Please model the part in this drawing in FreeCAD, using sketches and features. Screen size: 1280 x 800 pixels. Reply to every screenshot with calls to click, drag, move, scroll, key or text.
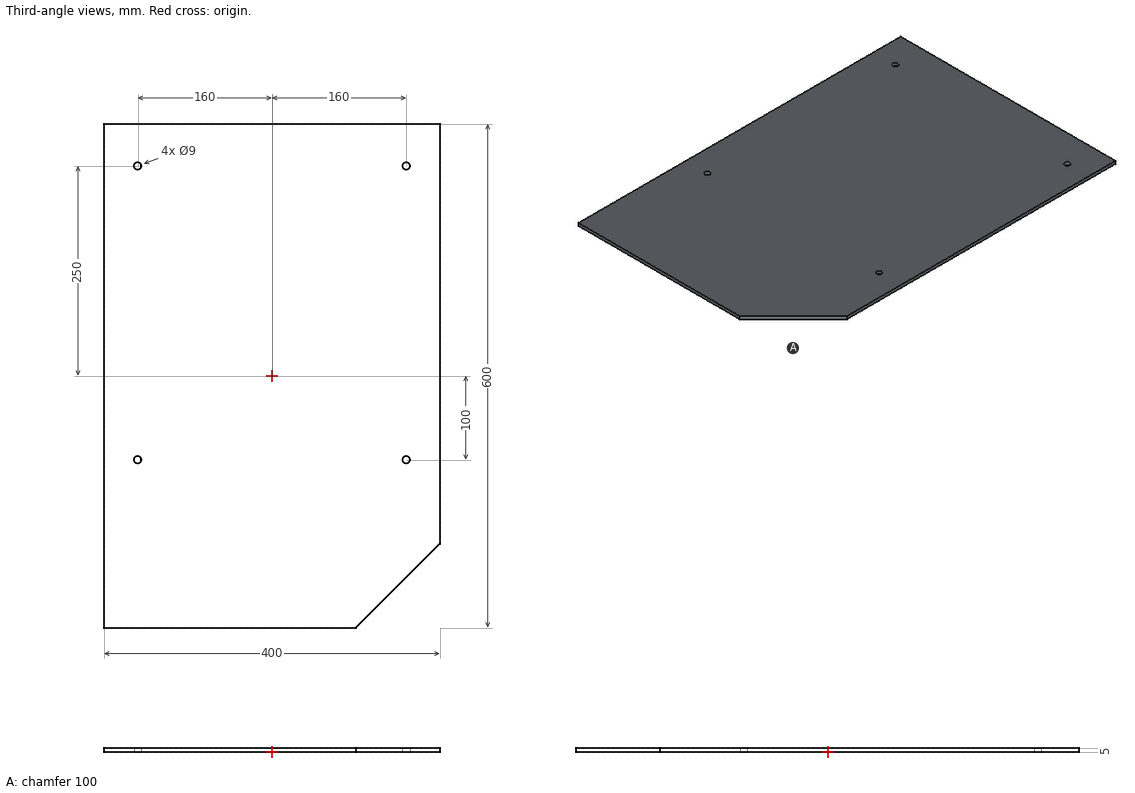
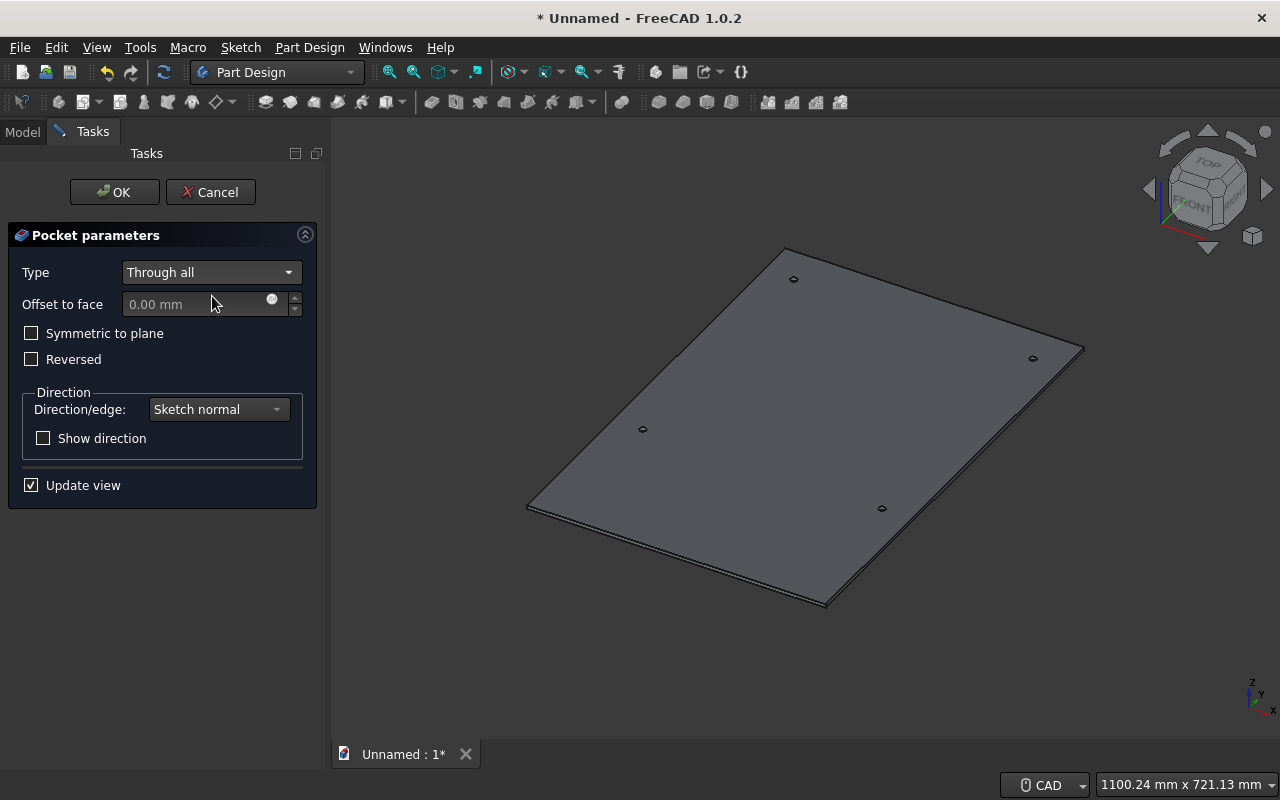
click(115, 192)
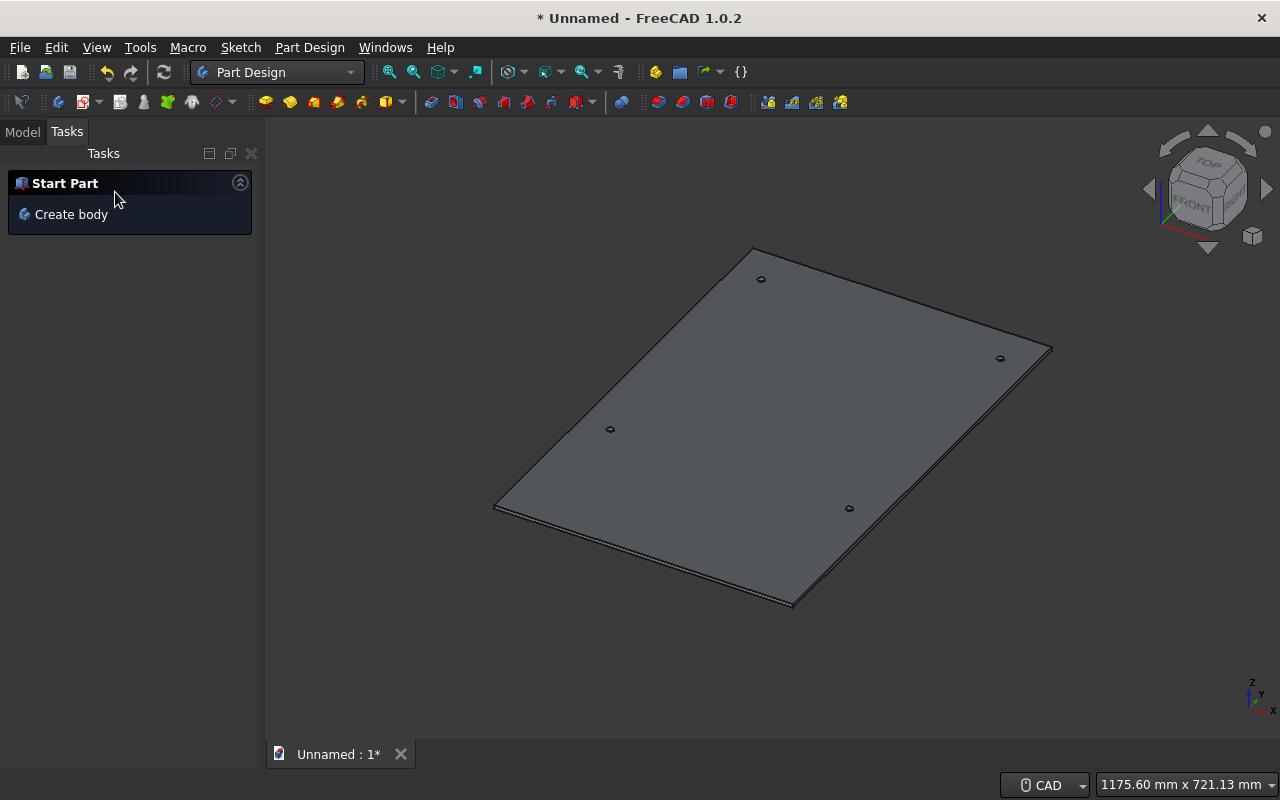
scroll(793, 605, up, 12)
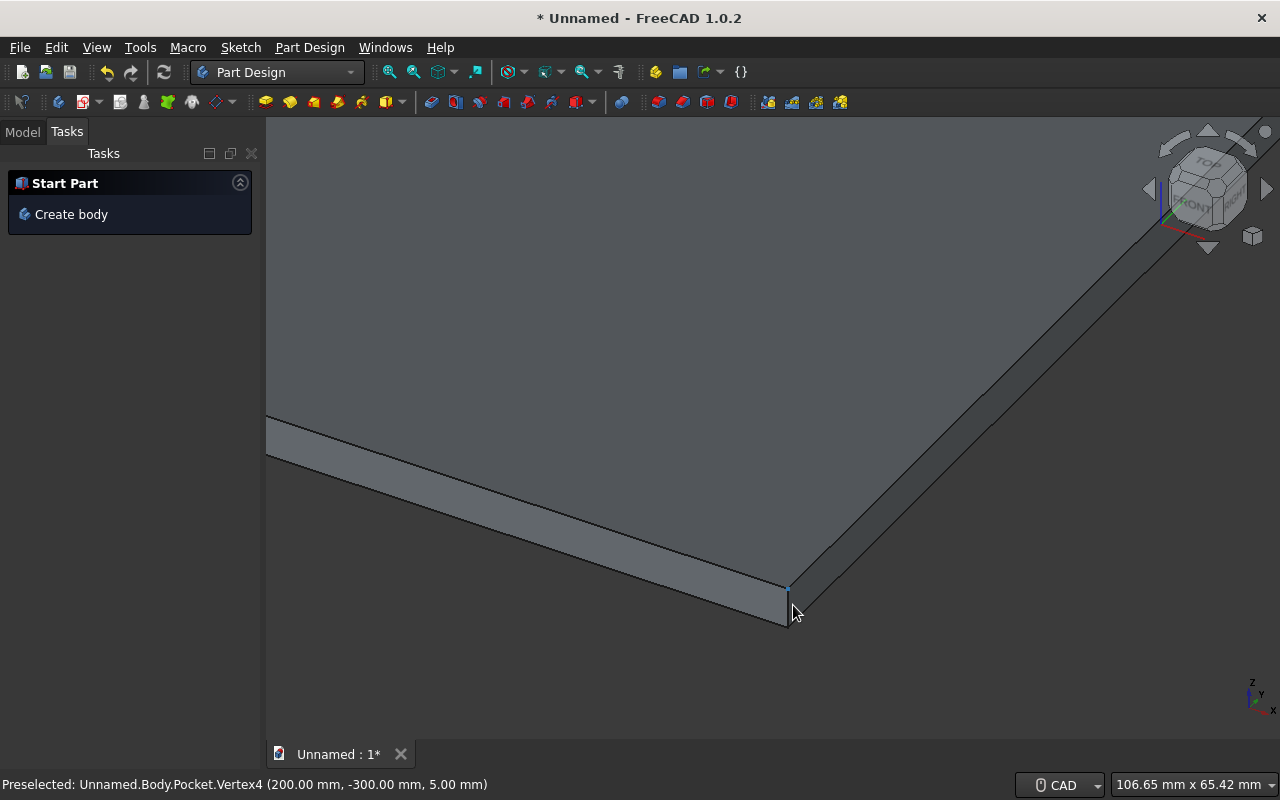
click(788, 607)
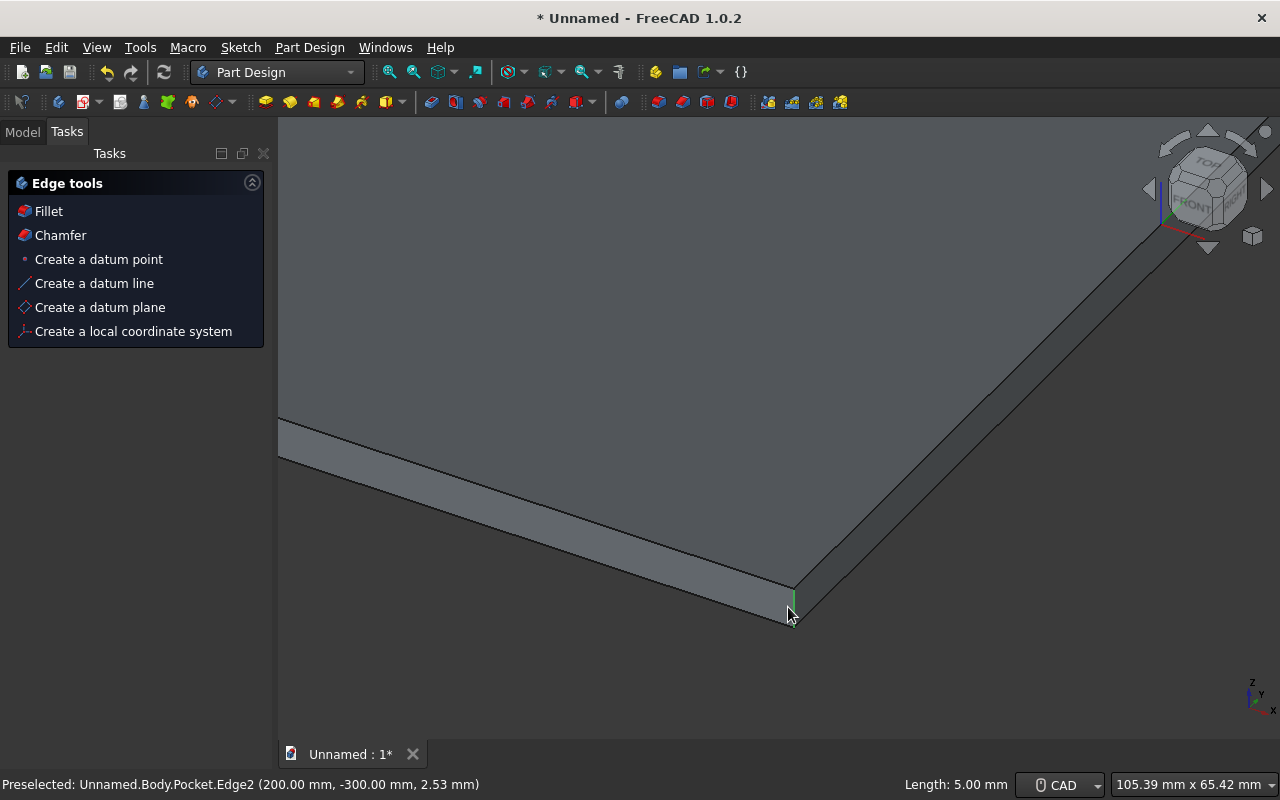
click(684, 102)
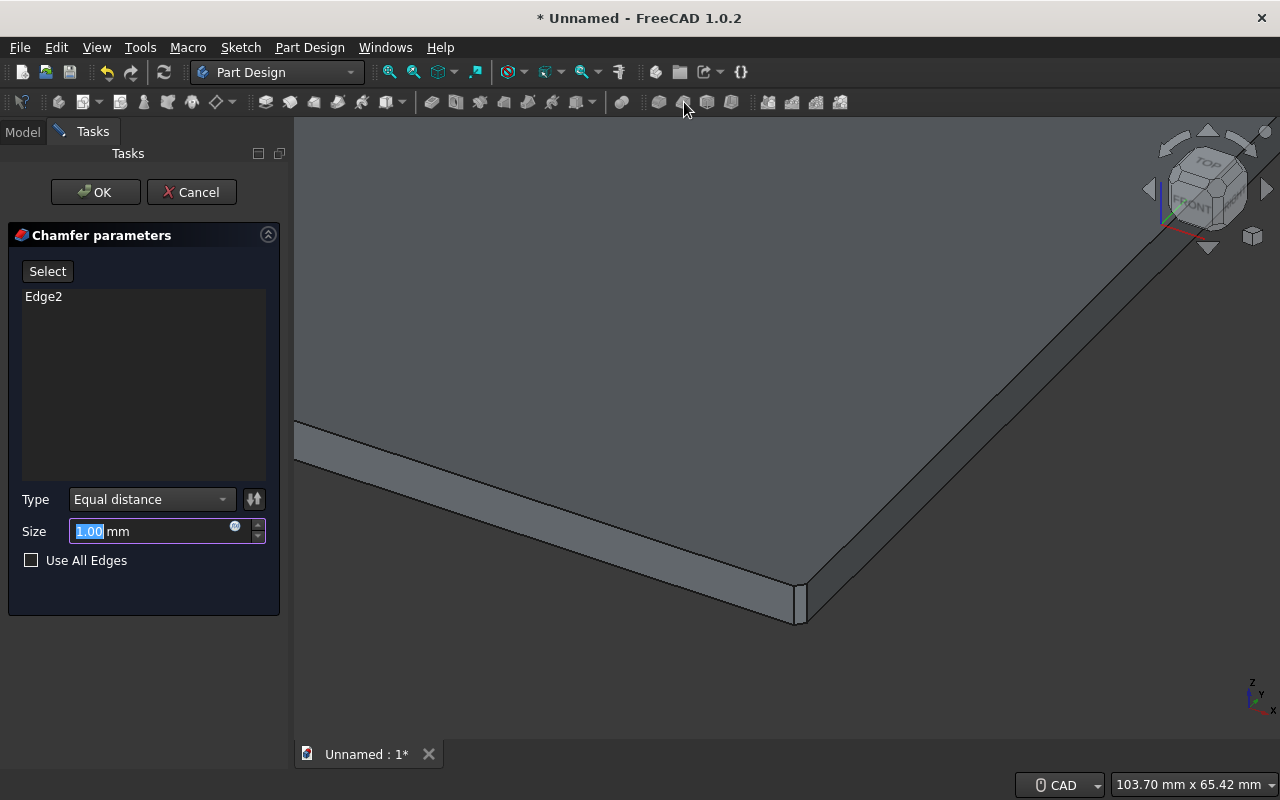
text(100)
key(Tab)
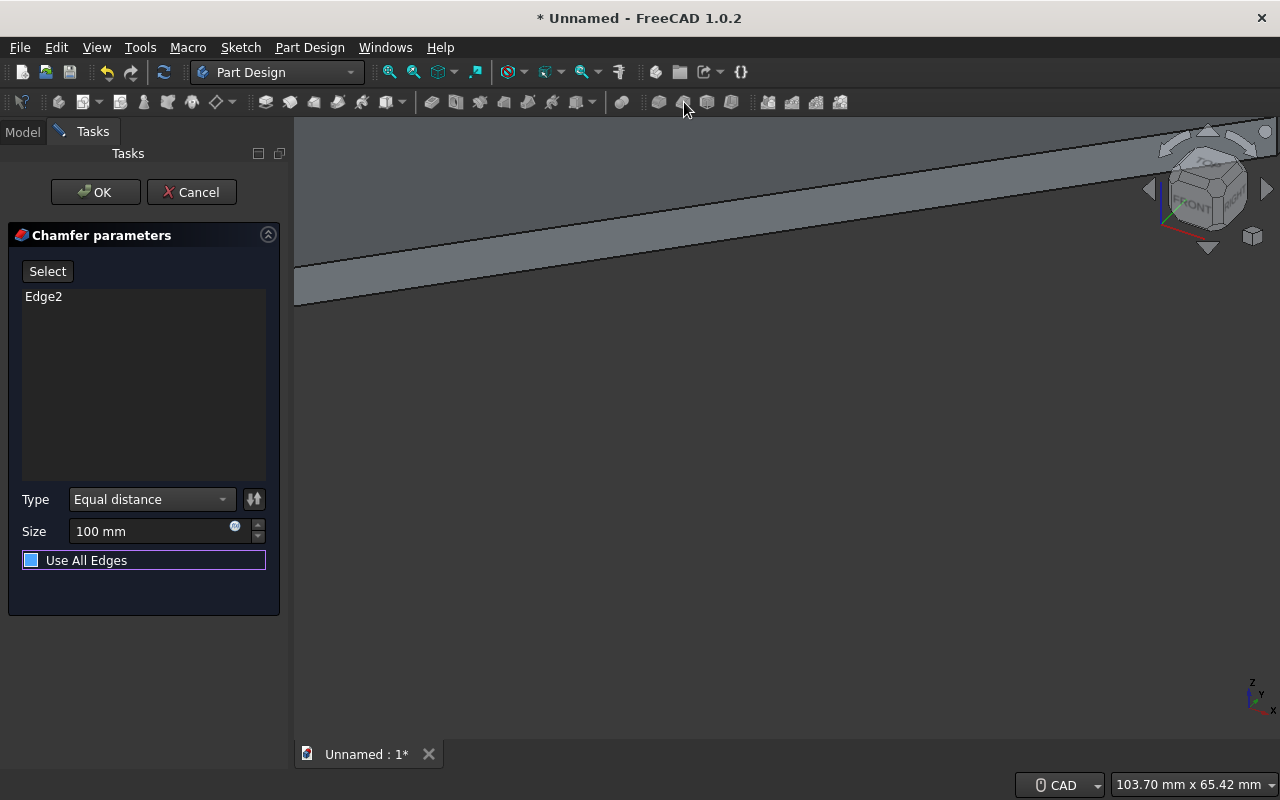
click(96, 192)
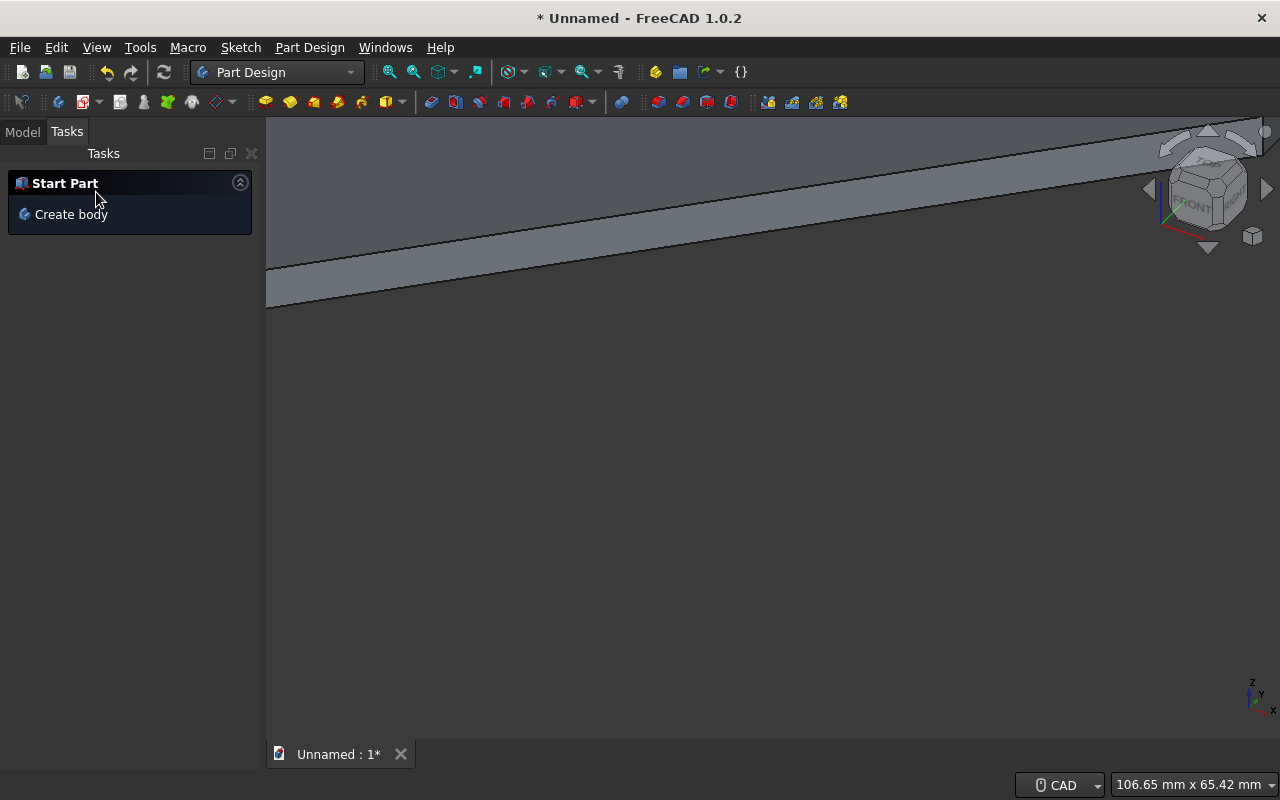
key(0)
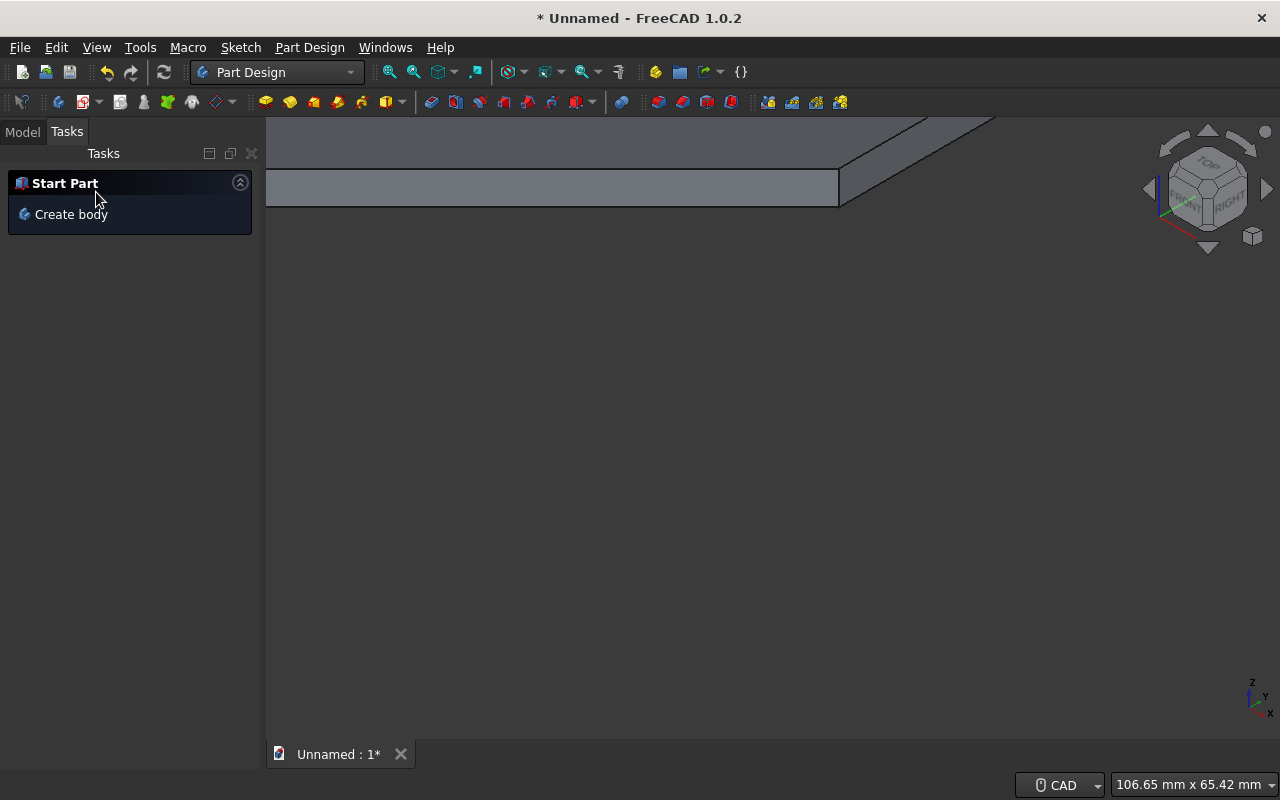
click(390, 72)